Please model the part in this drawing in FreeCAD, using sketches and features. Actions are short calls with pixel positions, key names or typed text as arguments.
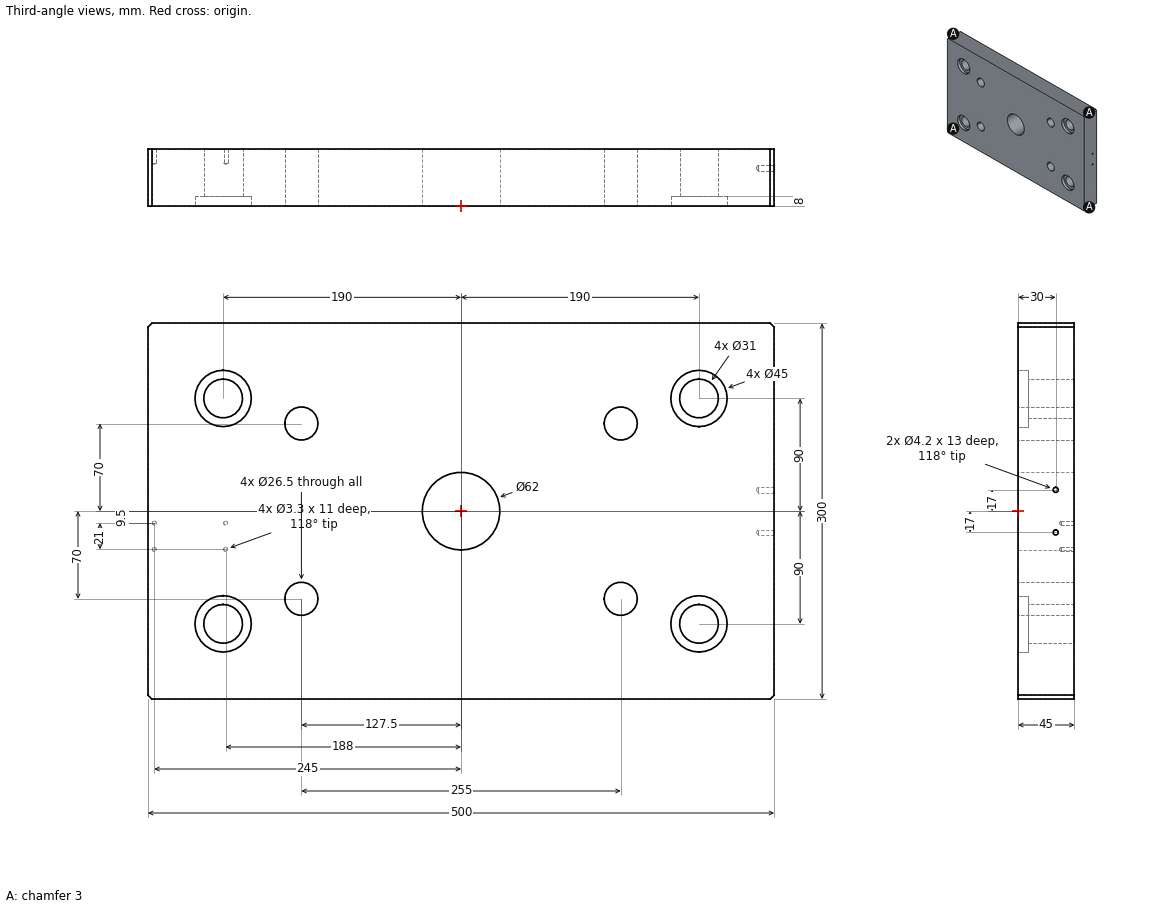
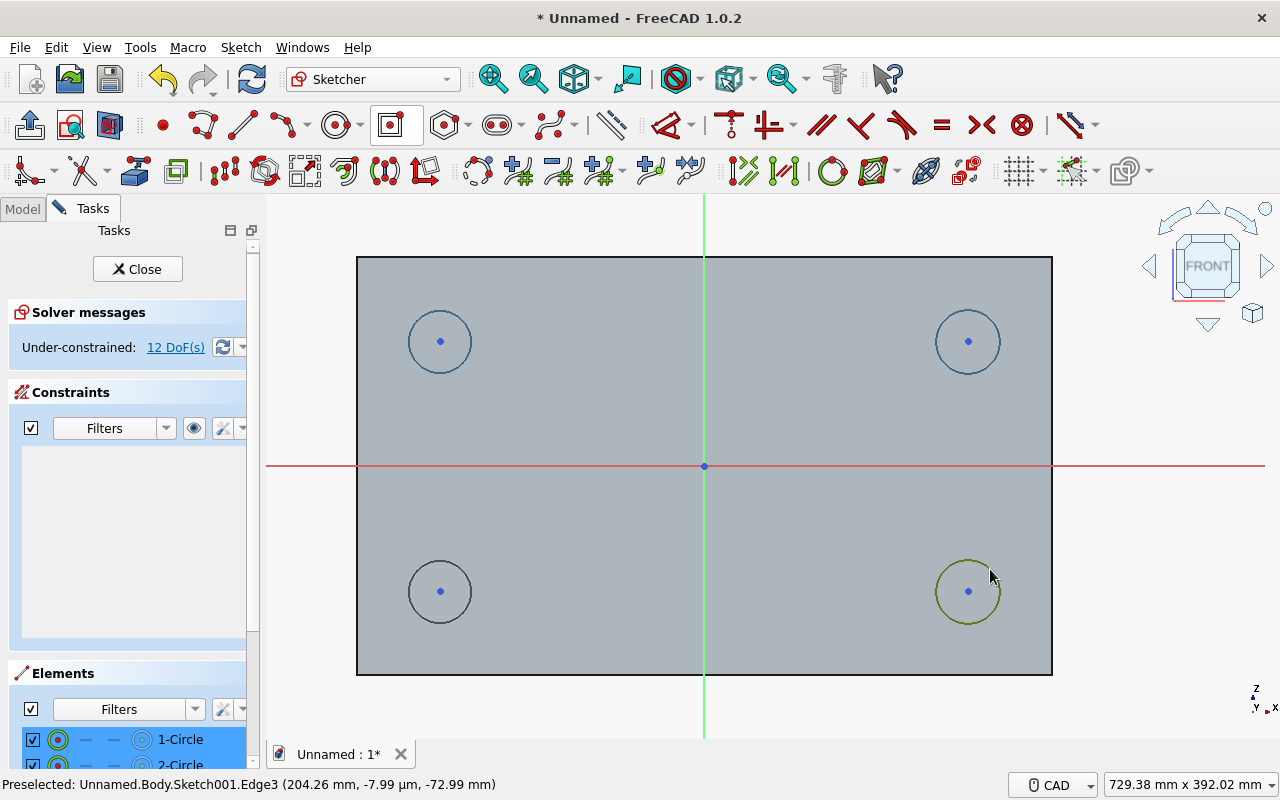
click(462, 570)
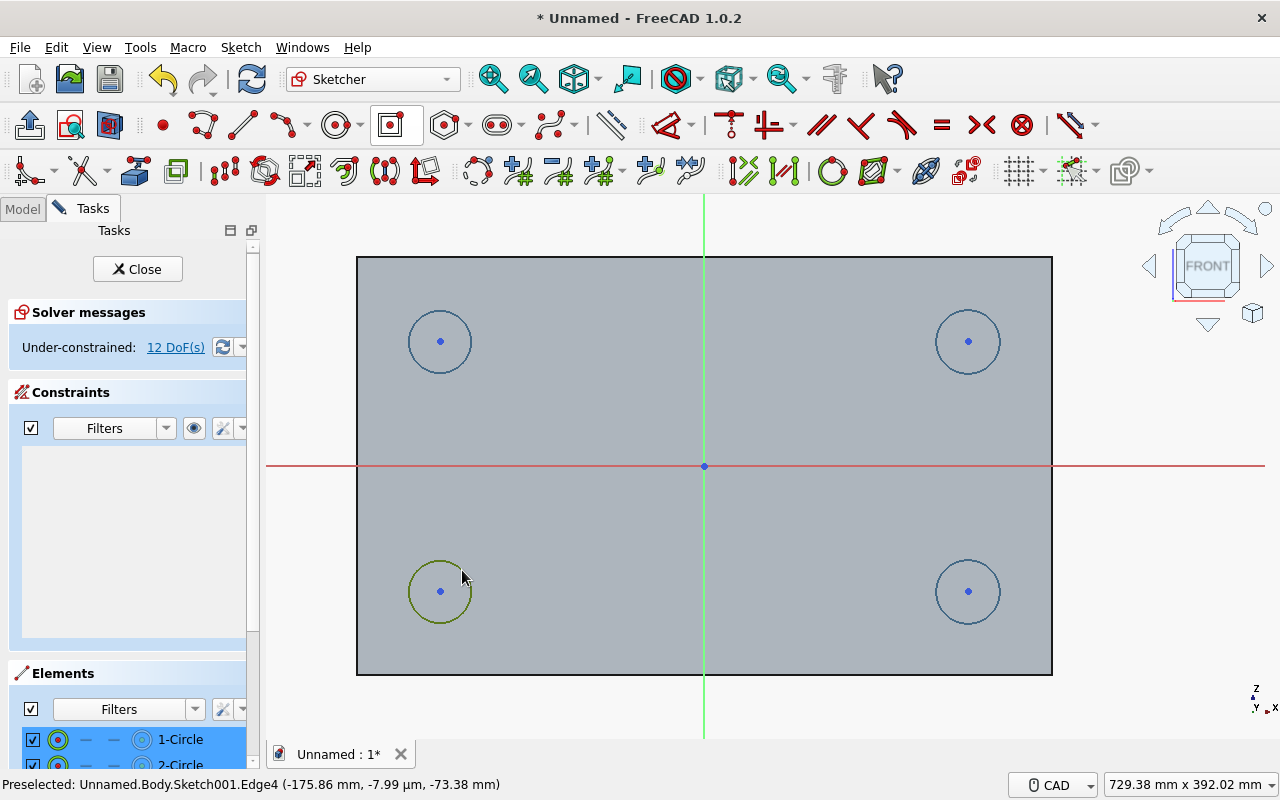
click(942, 126)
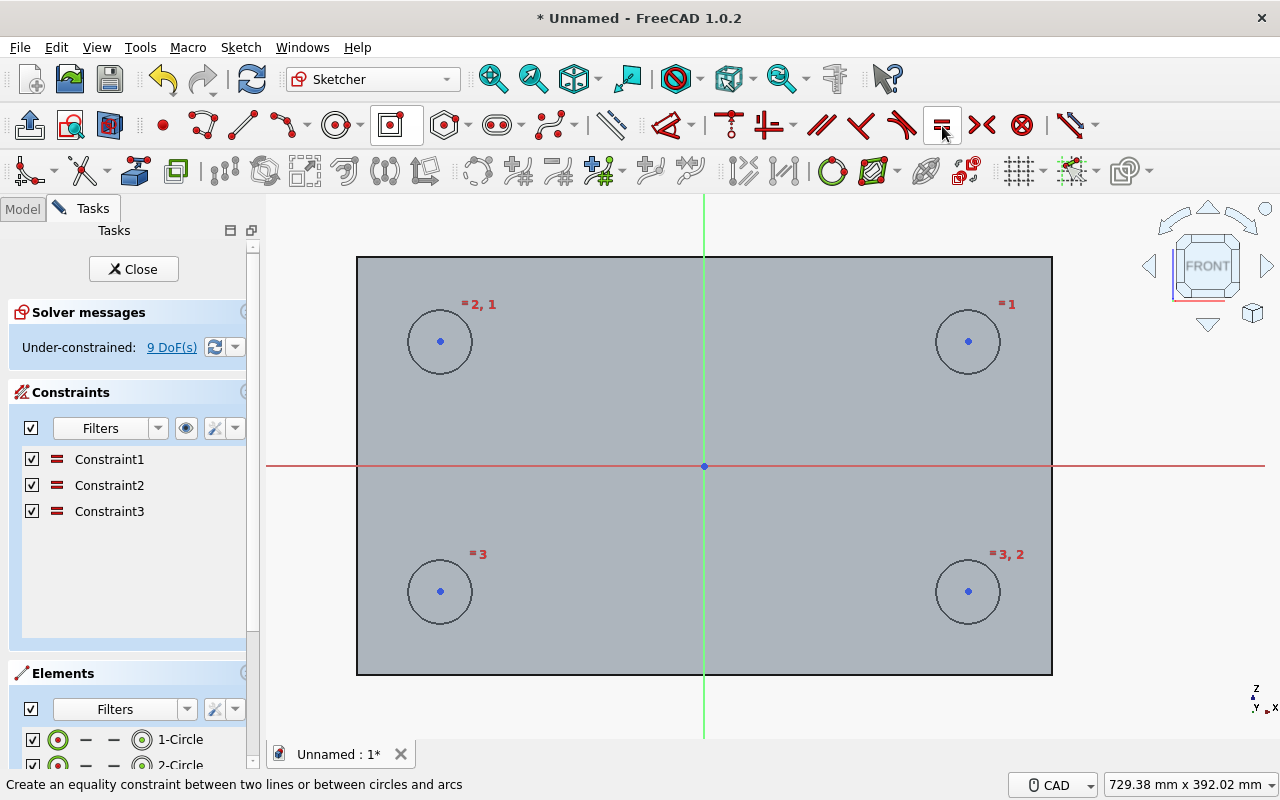
click(968, 342)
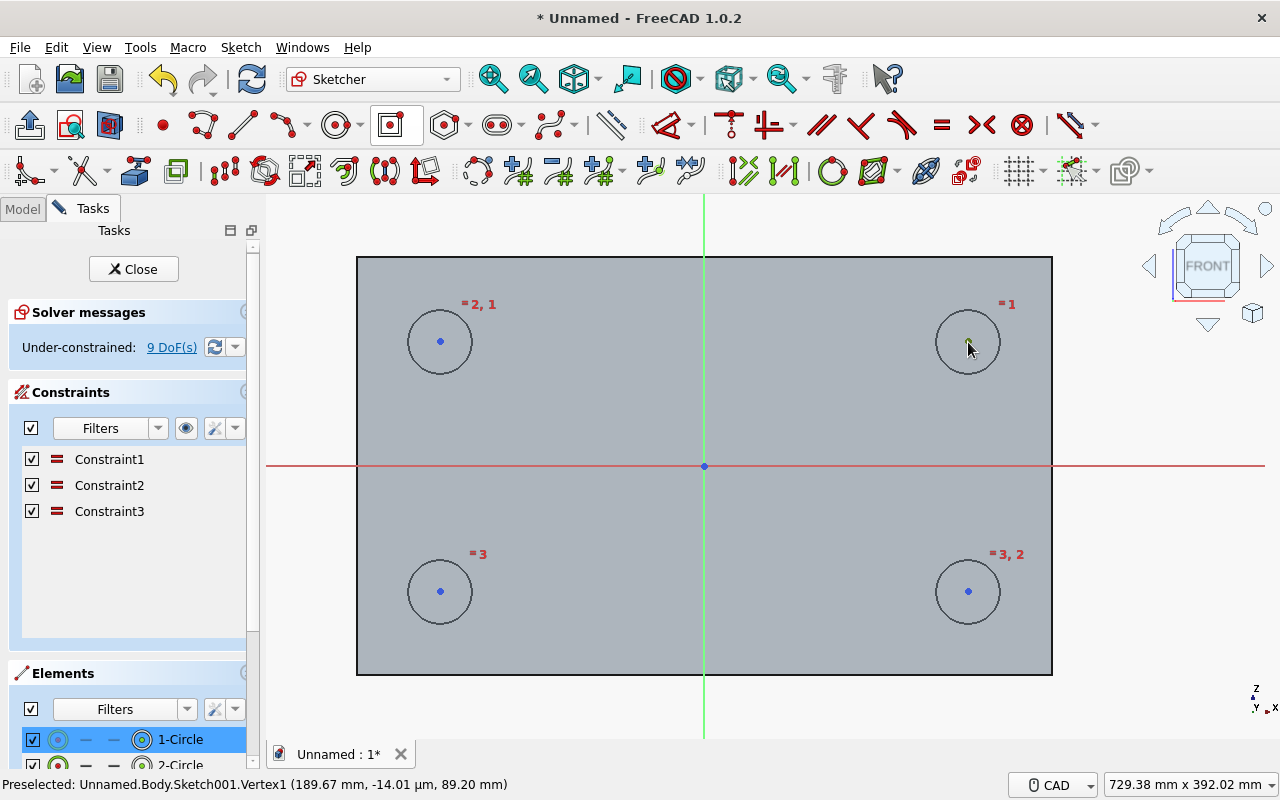
click(440, 342)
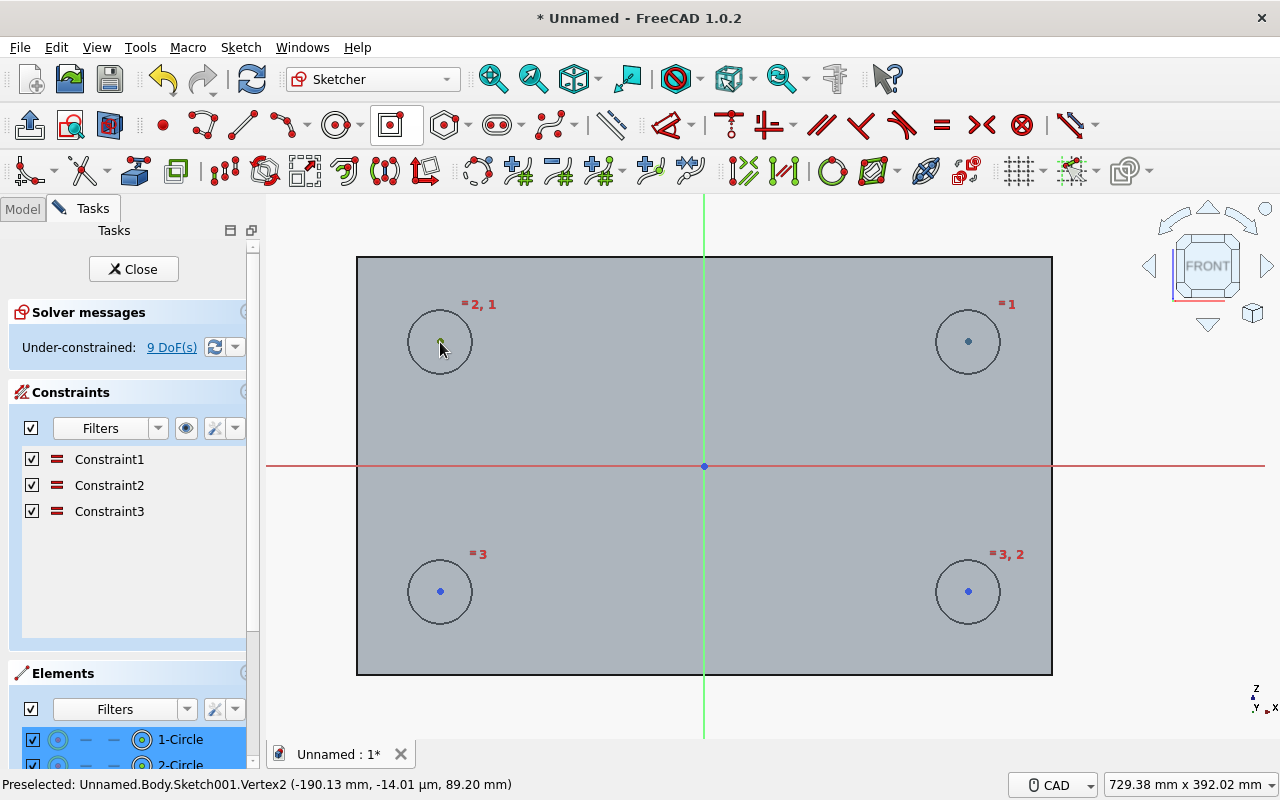
key(h)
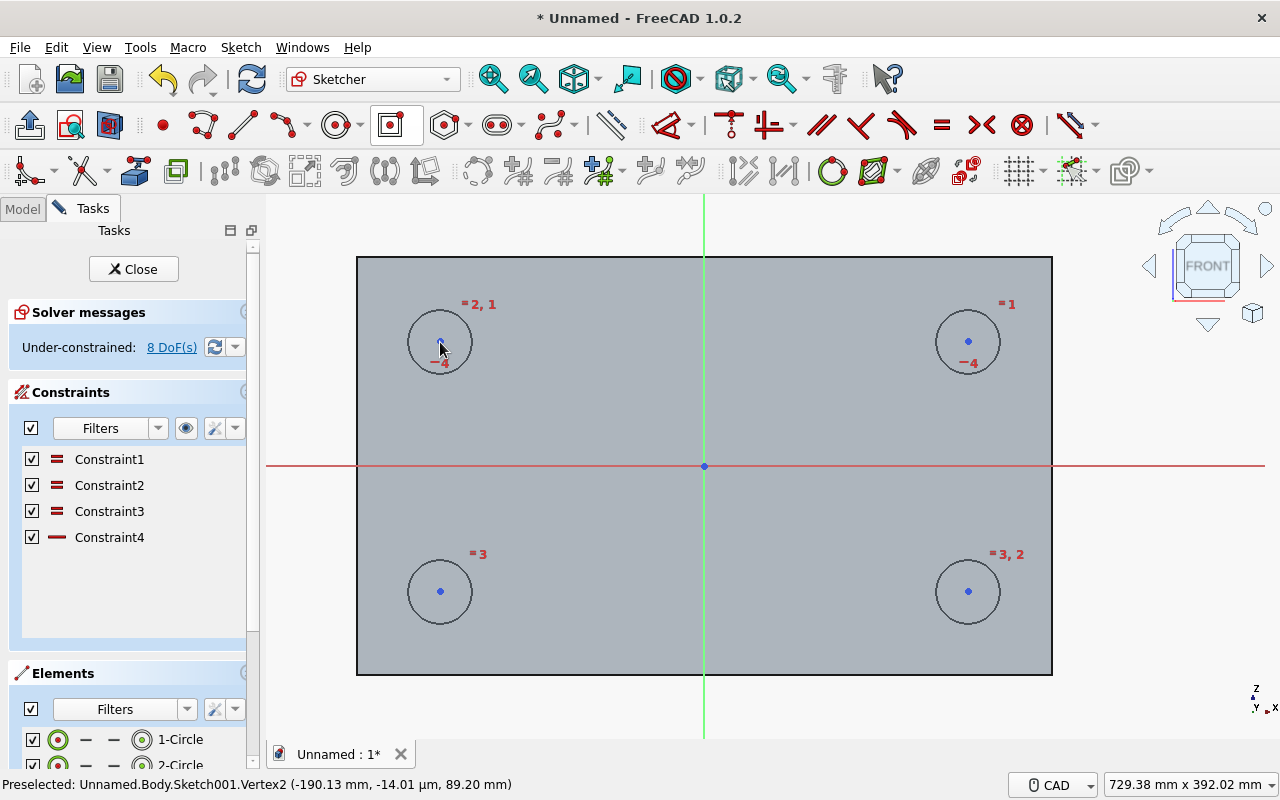
click(968, 342)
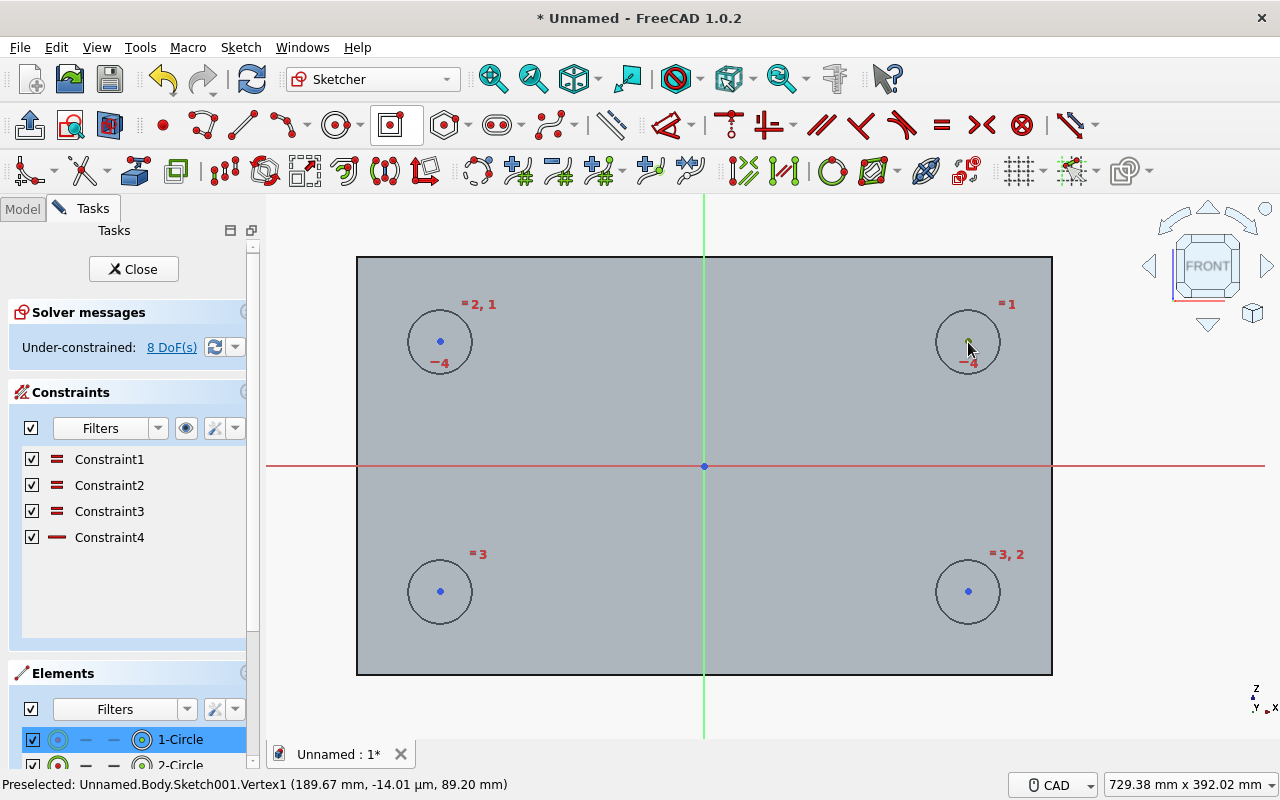
click(968, 592)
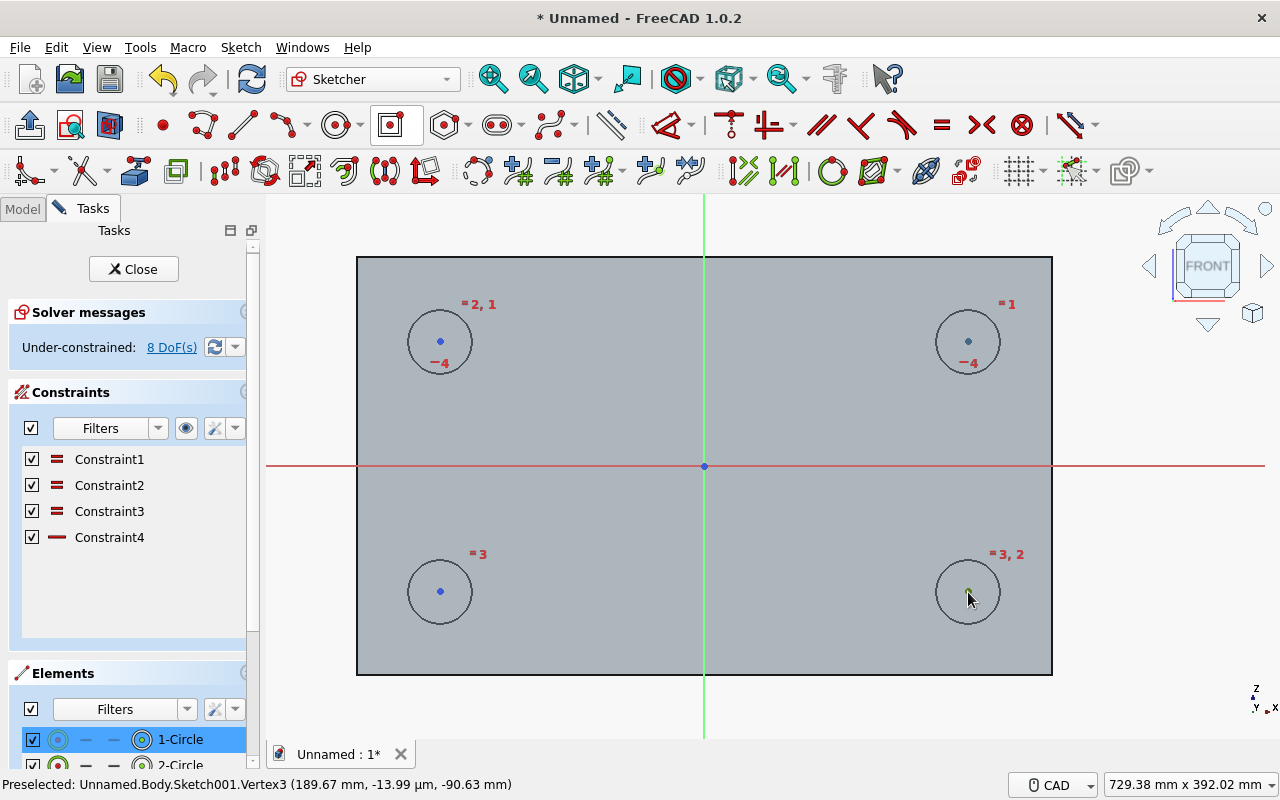
click(796, 126)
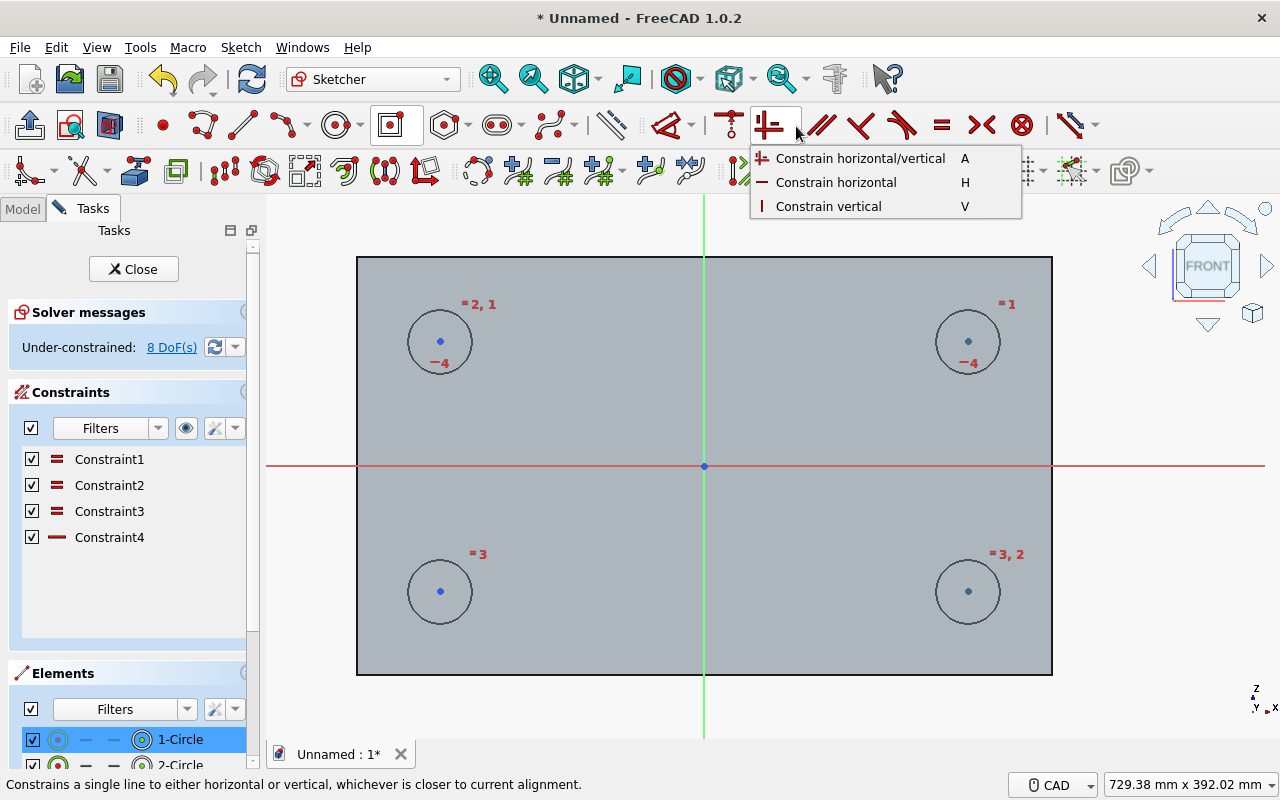
click(886, 206)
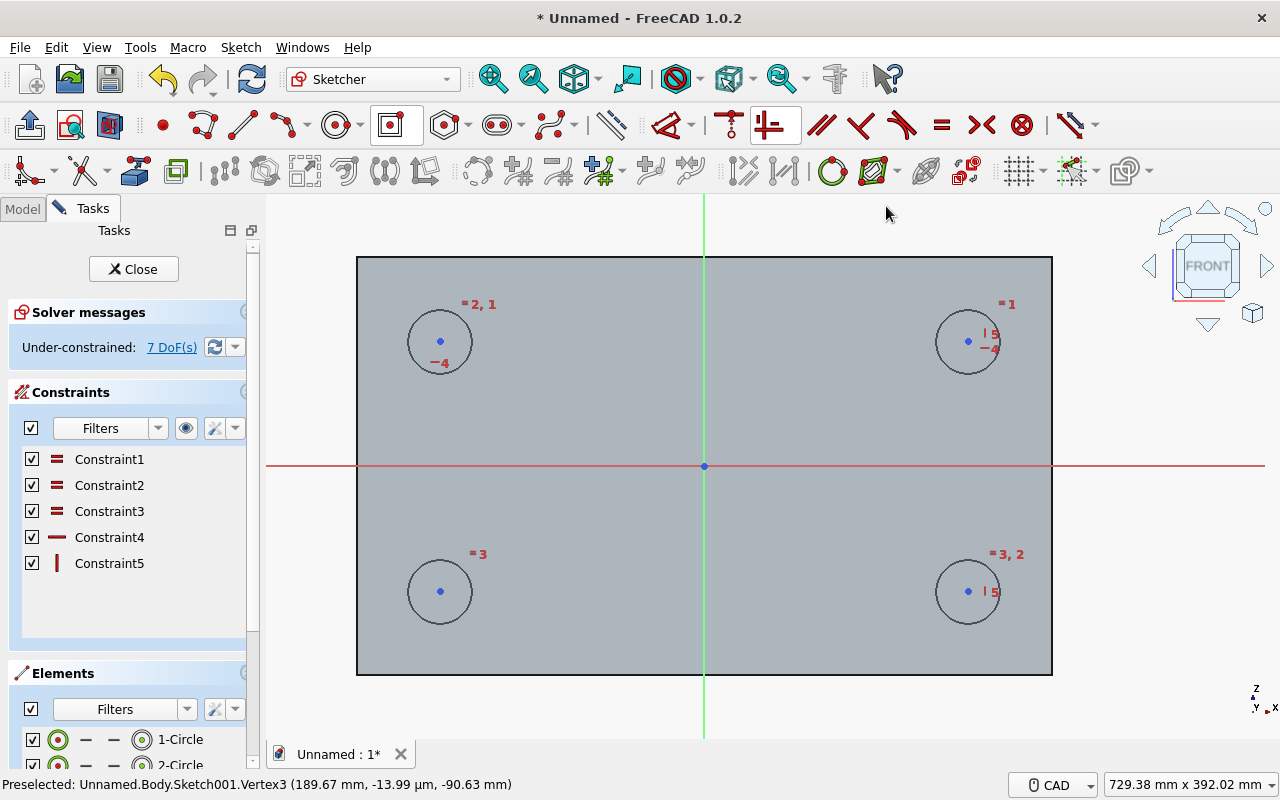
click(440, 342)